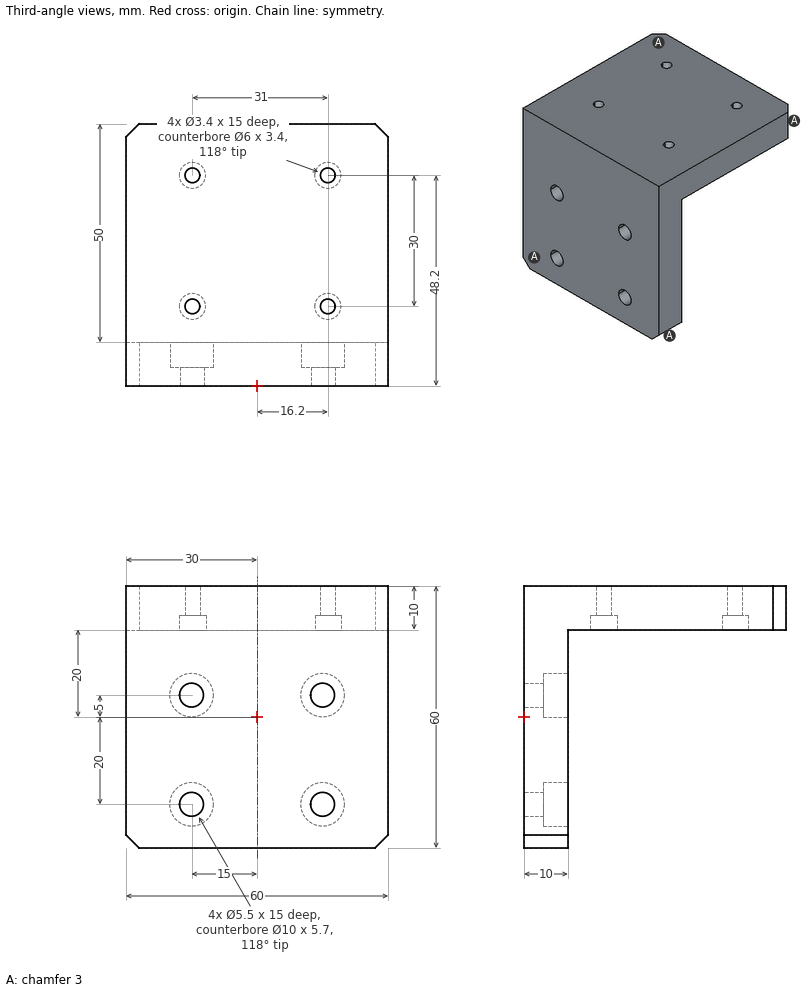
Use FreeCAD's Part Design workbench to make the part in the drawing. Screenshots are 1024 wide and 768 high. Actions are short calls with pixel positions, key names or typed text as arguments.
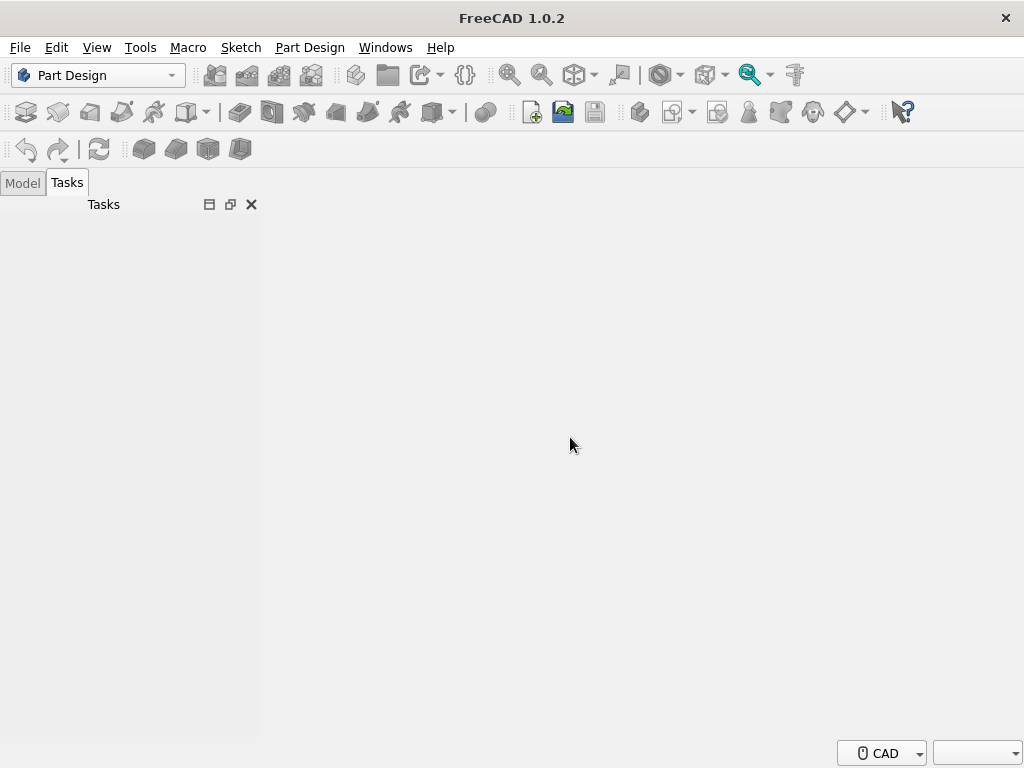
key(ctrl+n)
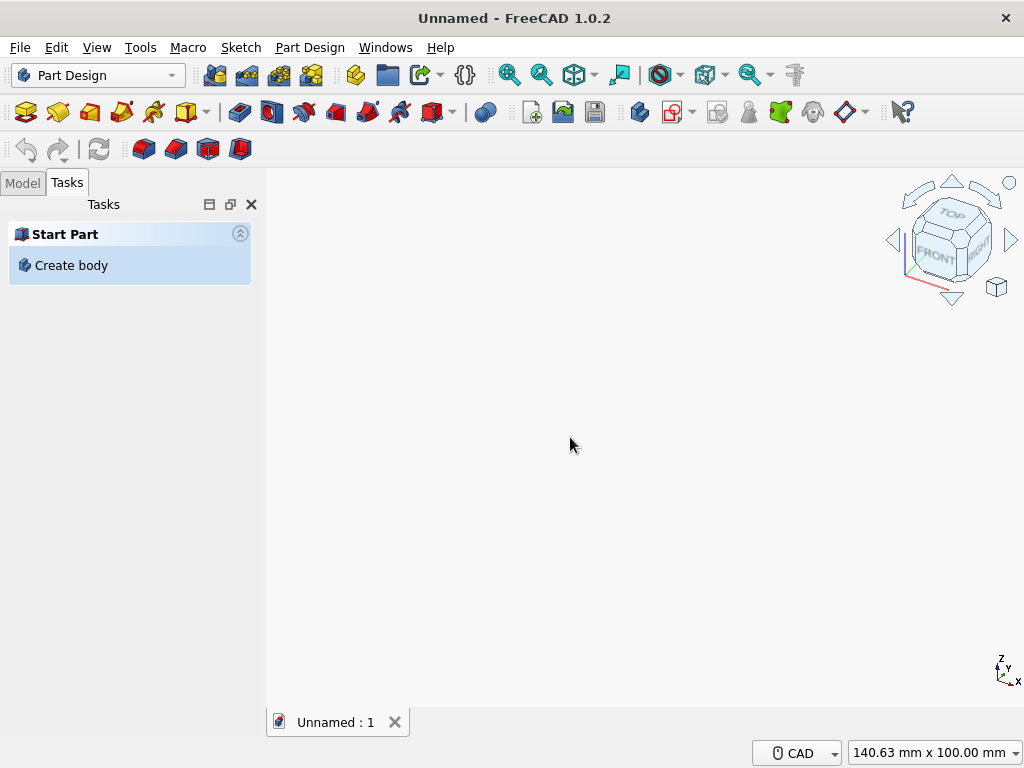
click(672, 112)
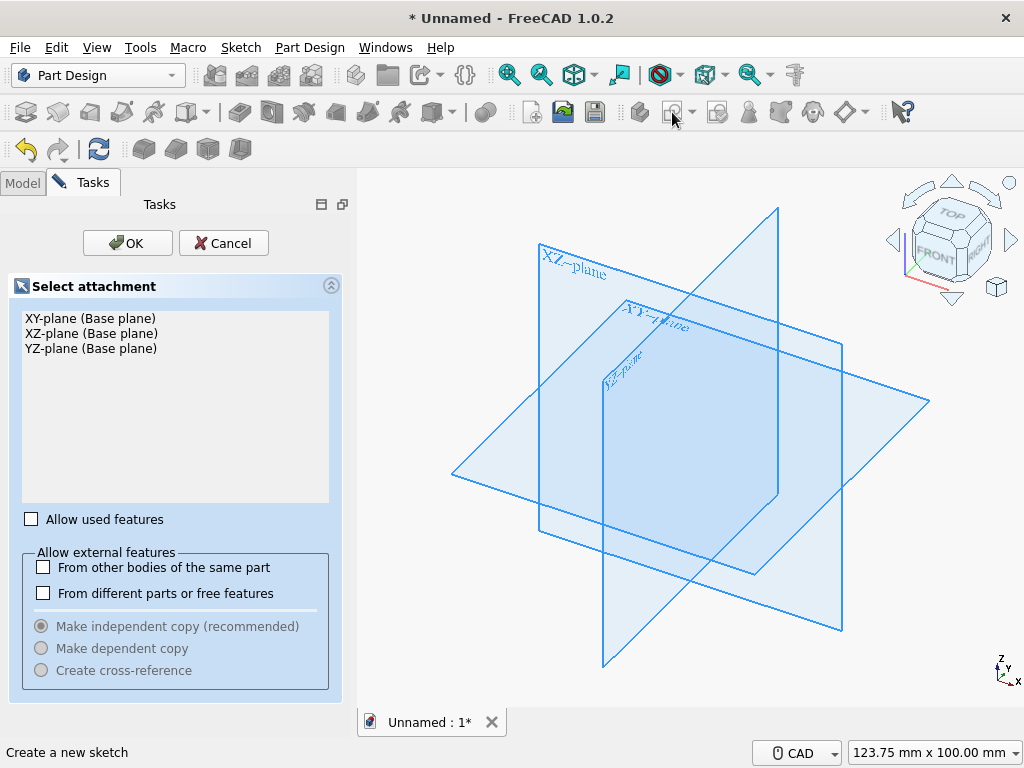
click(82, 334)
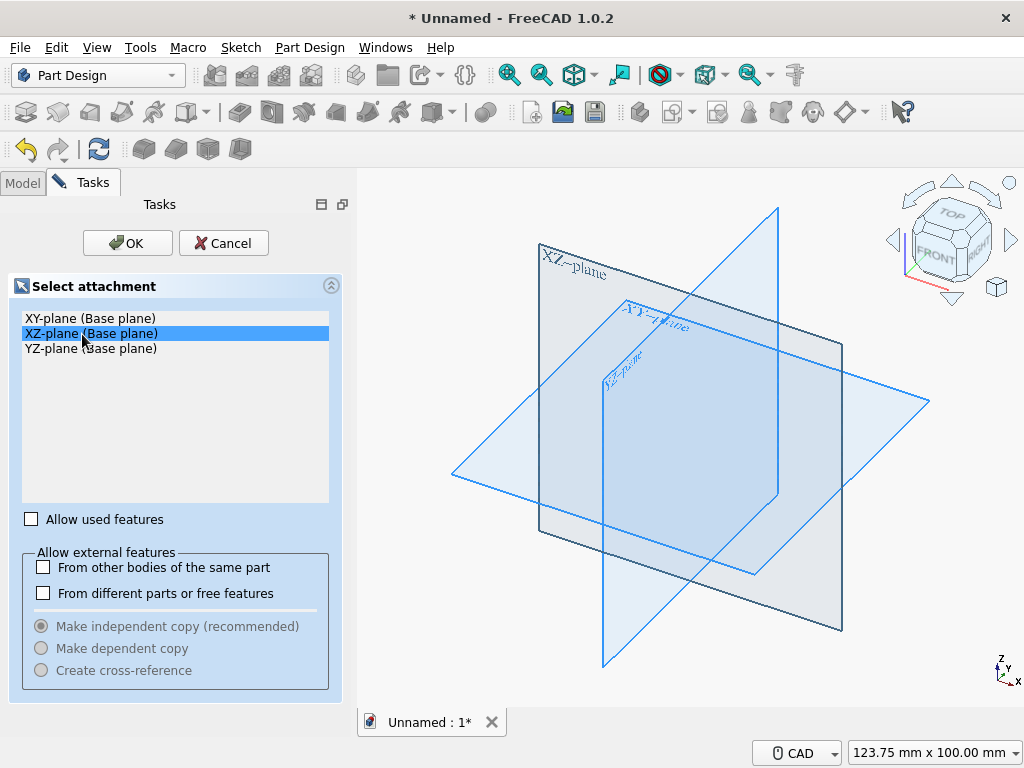
click(128, 243)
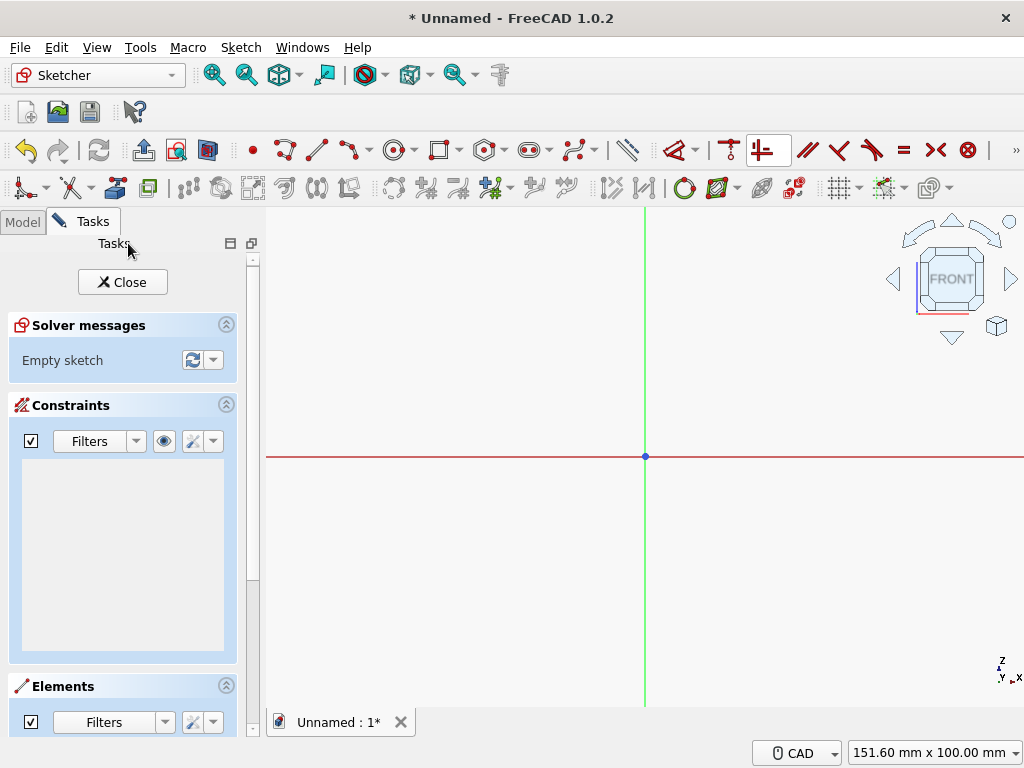
key(g)
key(v)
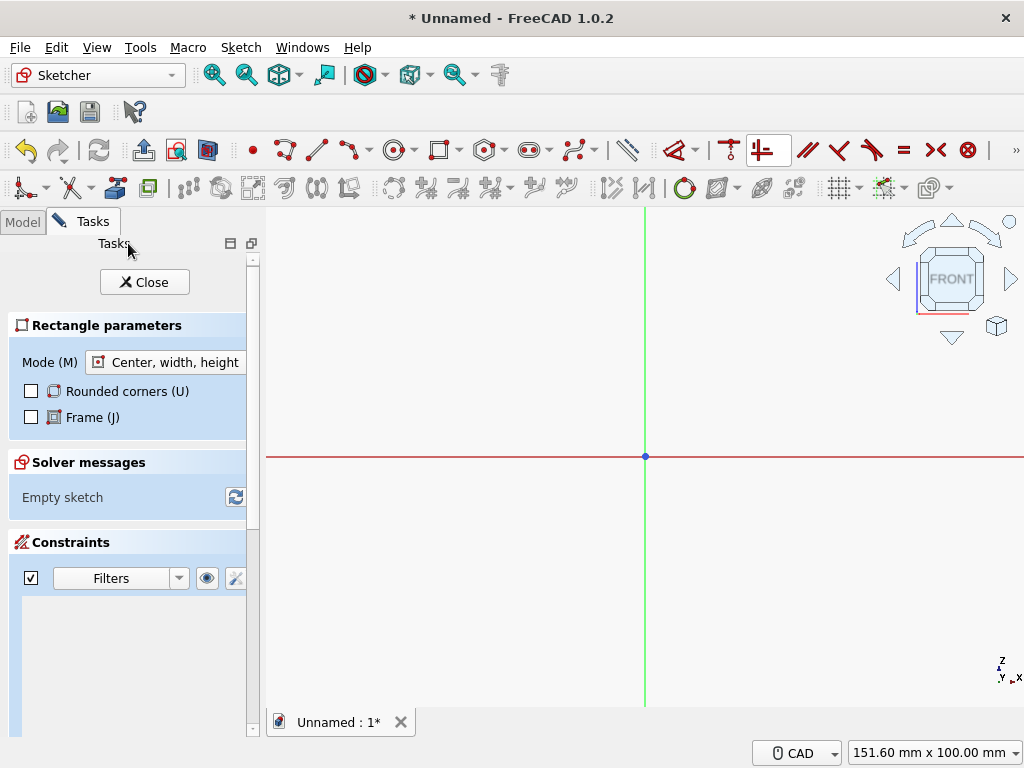
click(645, 457)
move(795, 307)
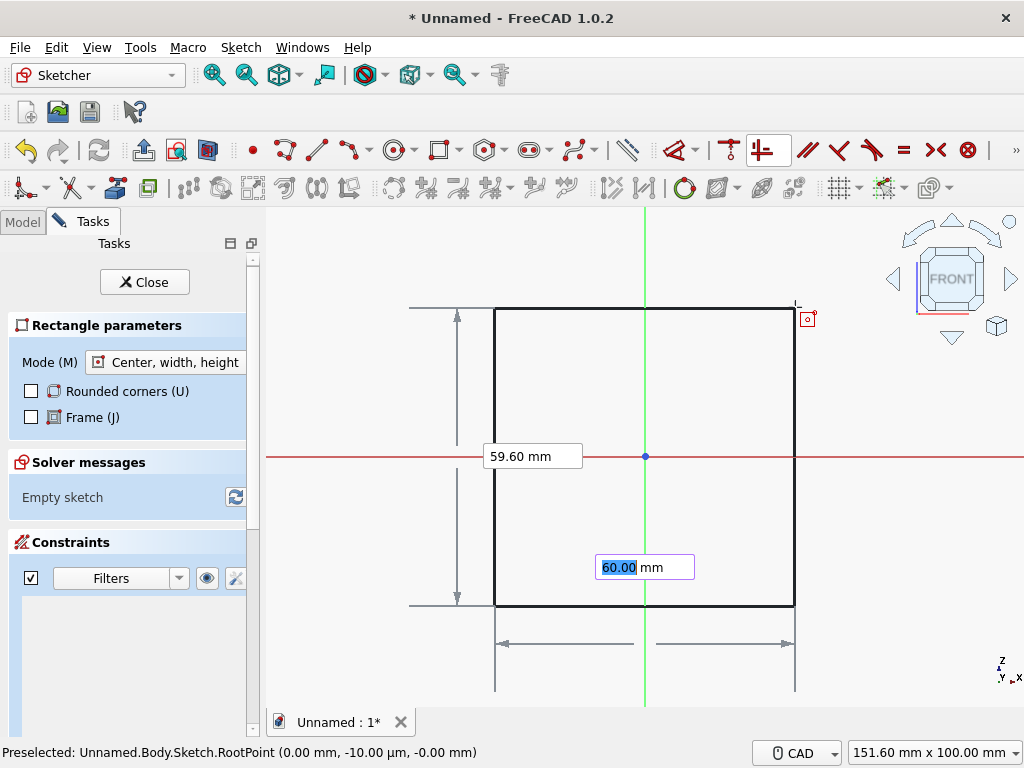
text(60)
key(Tab)
text(60)
key(Return)
key(Escape)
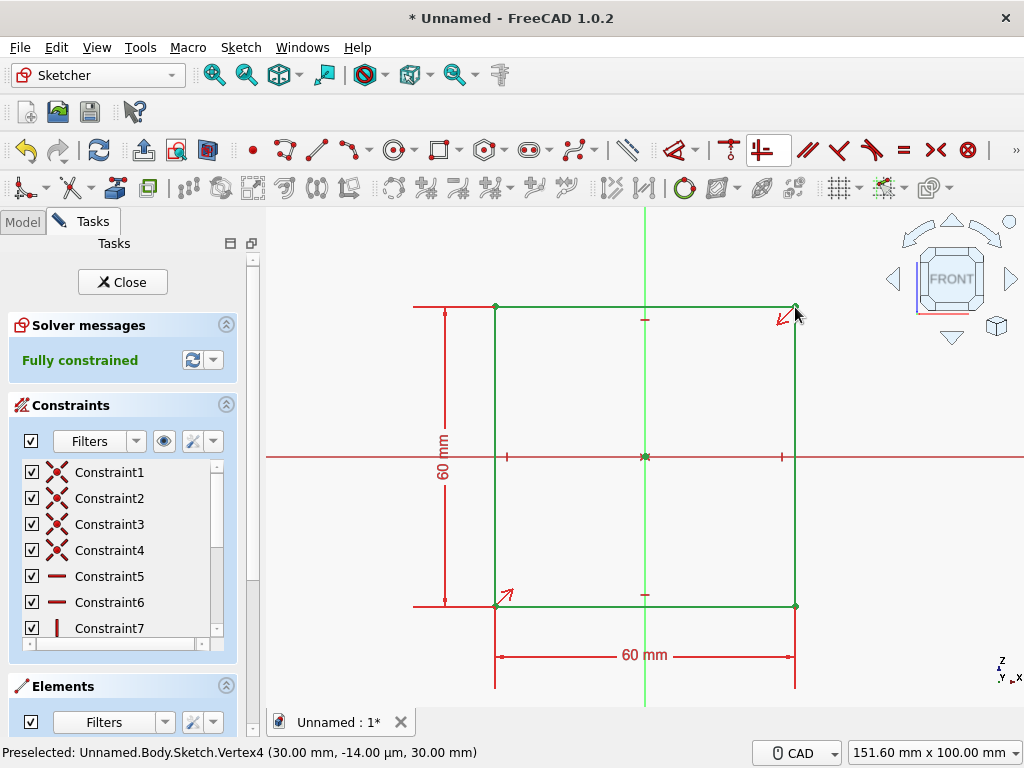
click(123, 282)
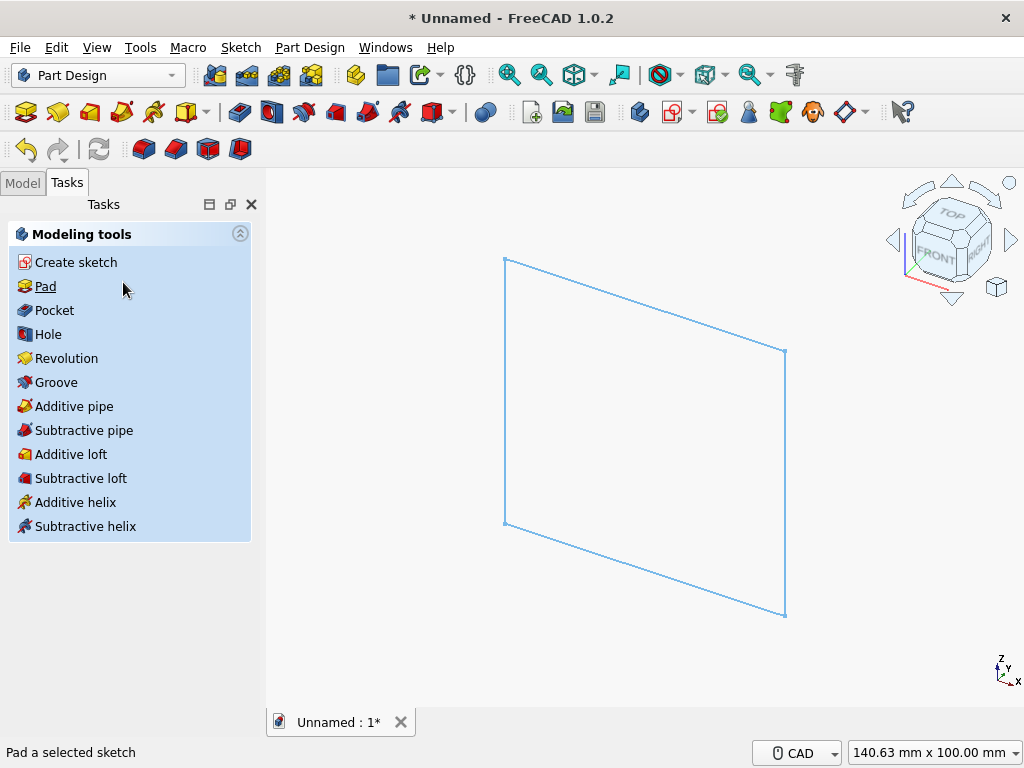
click(26, 112)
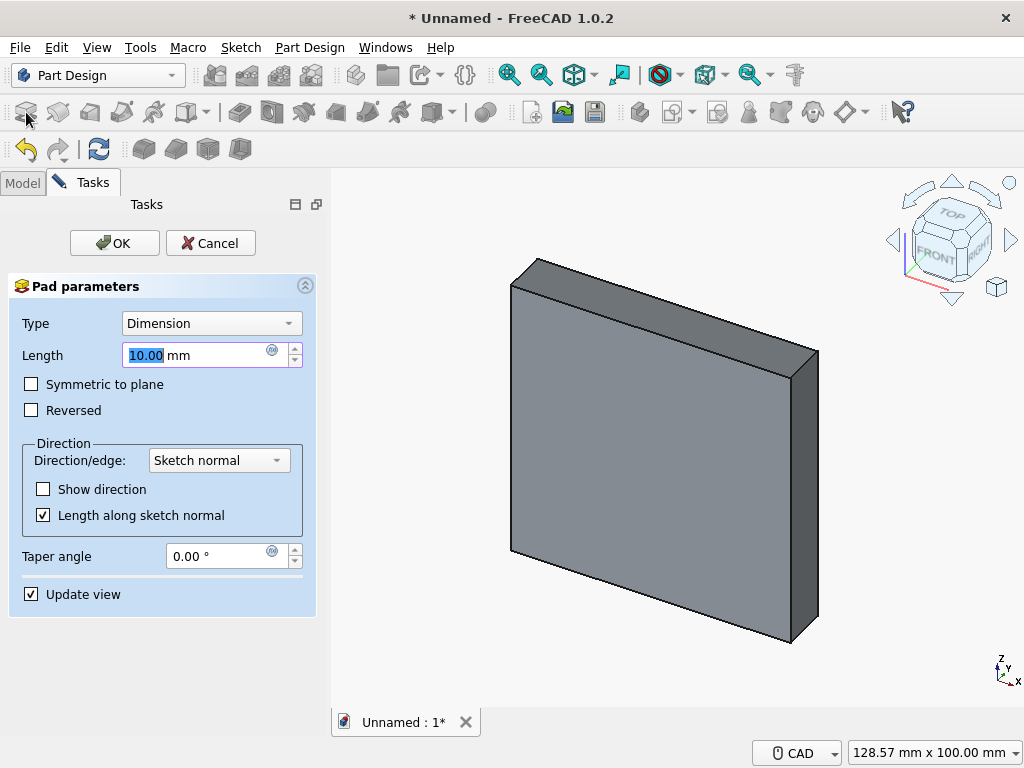
text(10)
key(Tab)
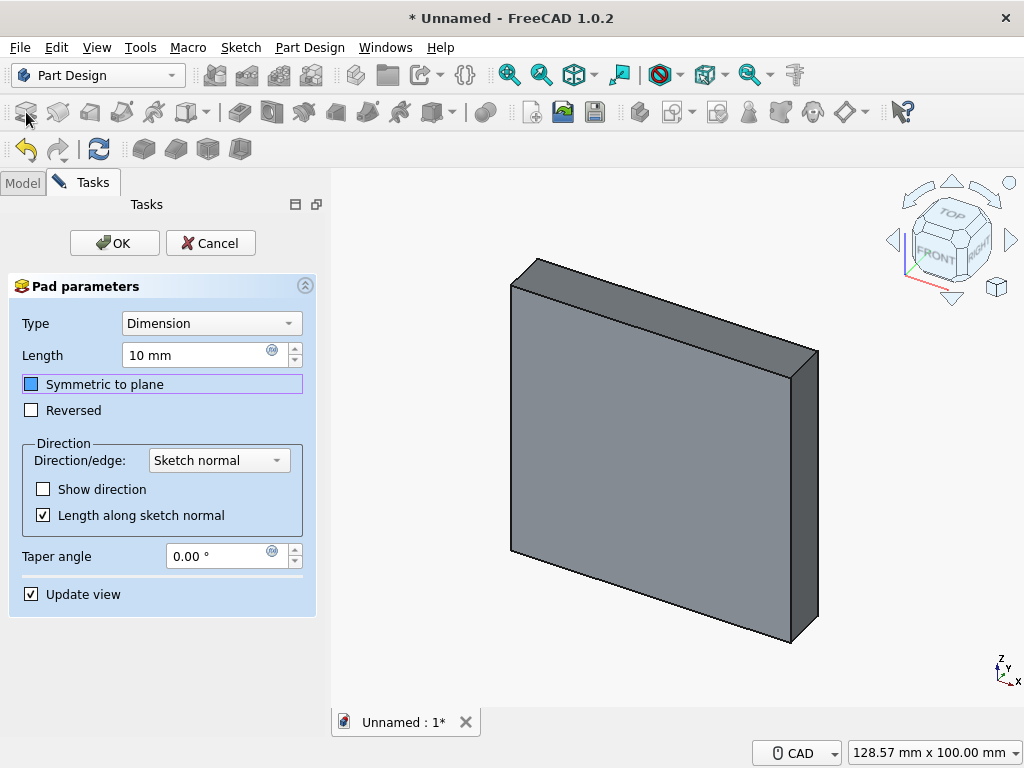
click(30, 410)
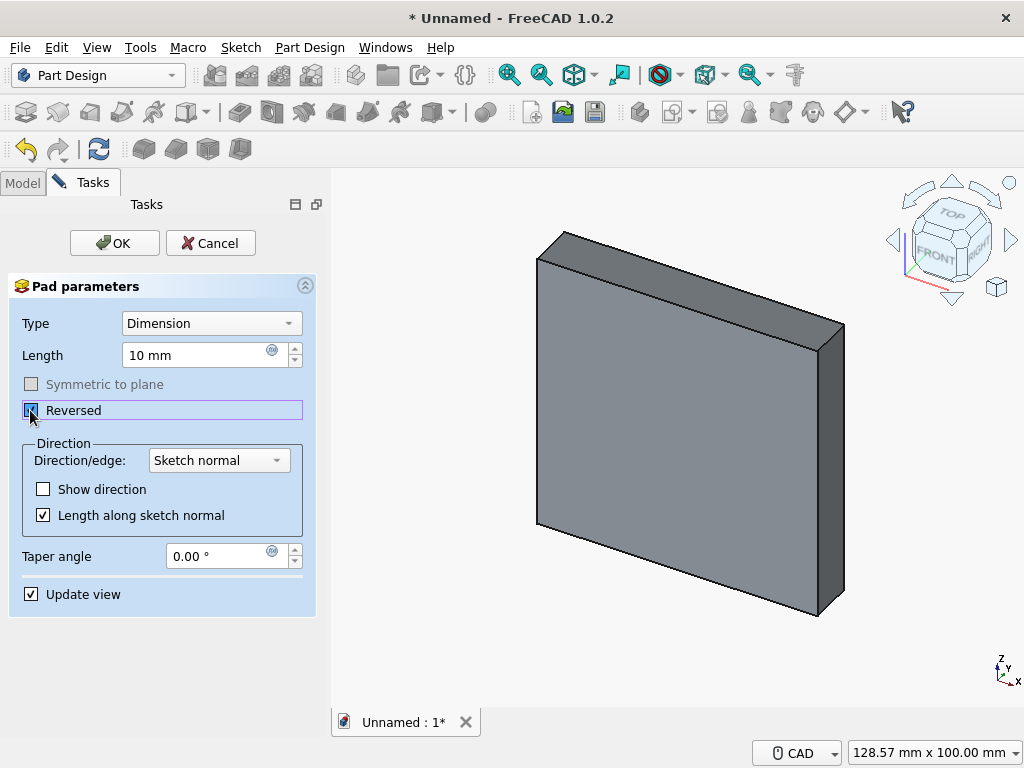
click(115, 243)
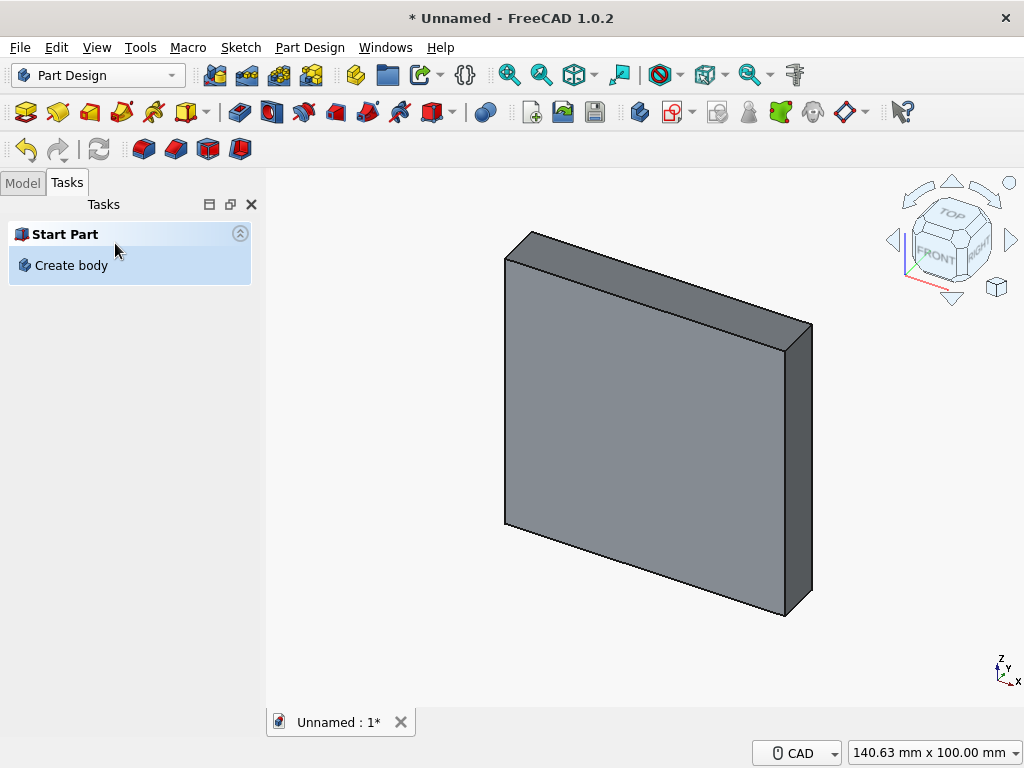
key(4)